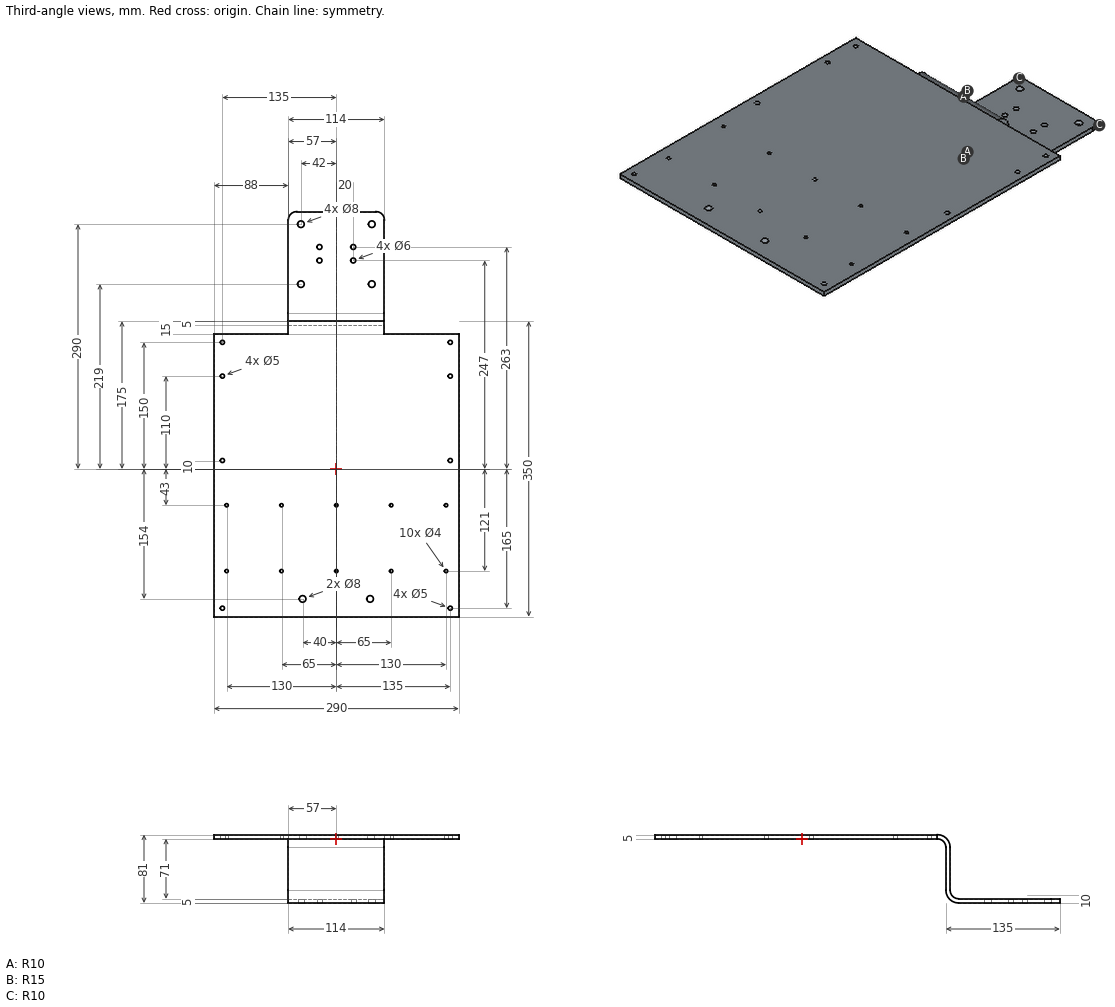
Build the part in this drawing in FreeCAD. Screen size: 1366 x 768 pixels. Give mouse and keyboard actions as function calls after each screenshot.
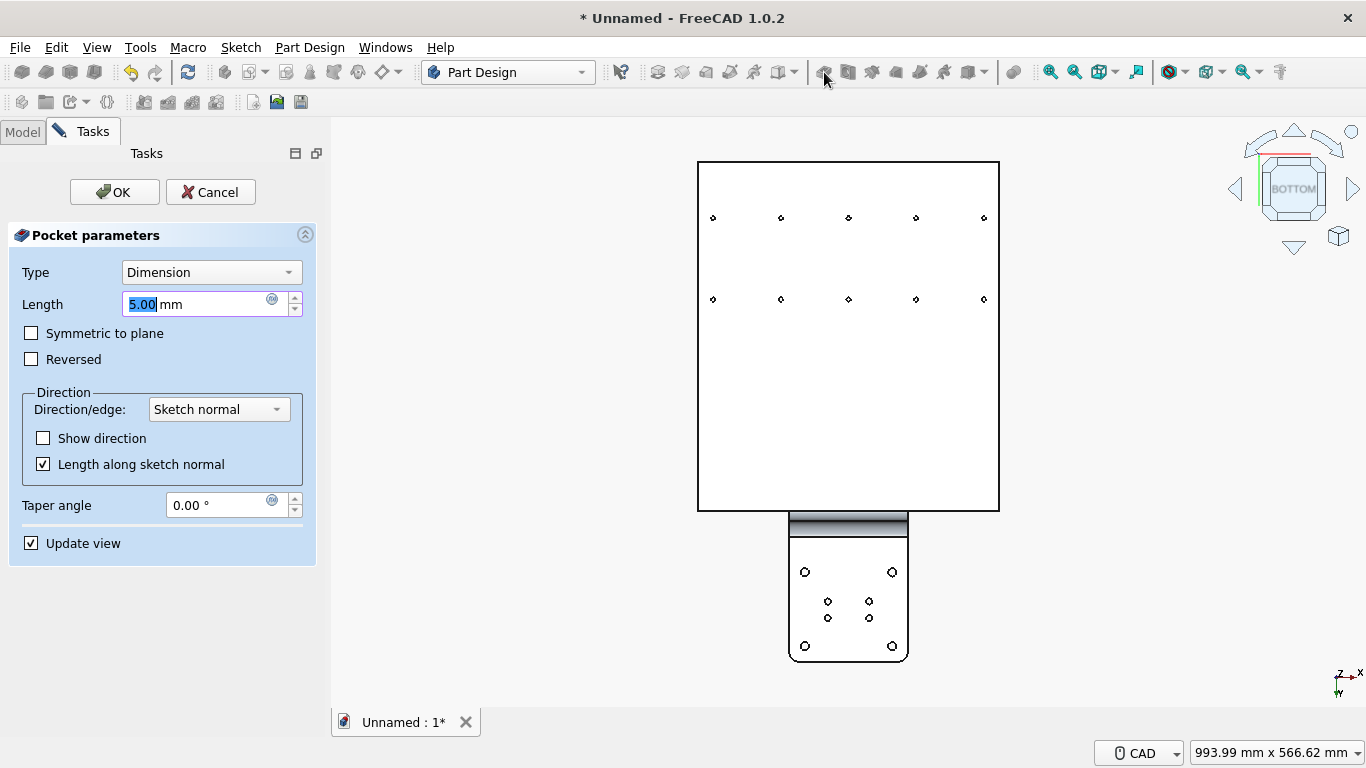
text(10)
key(Tab)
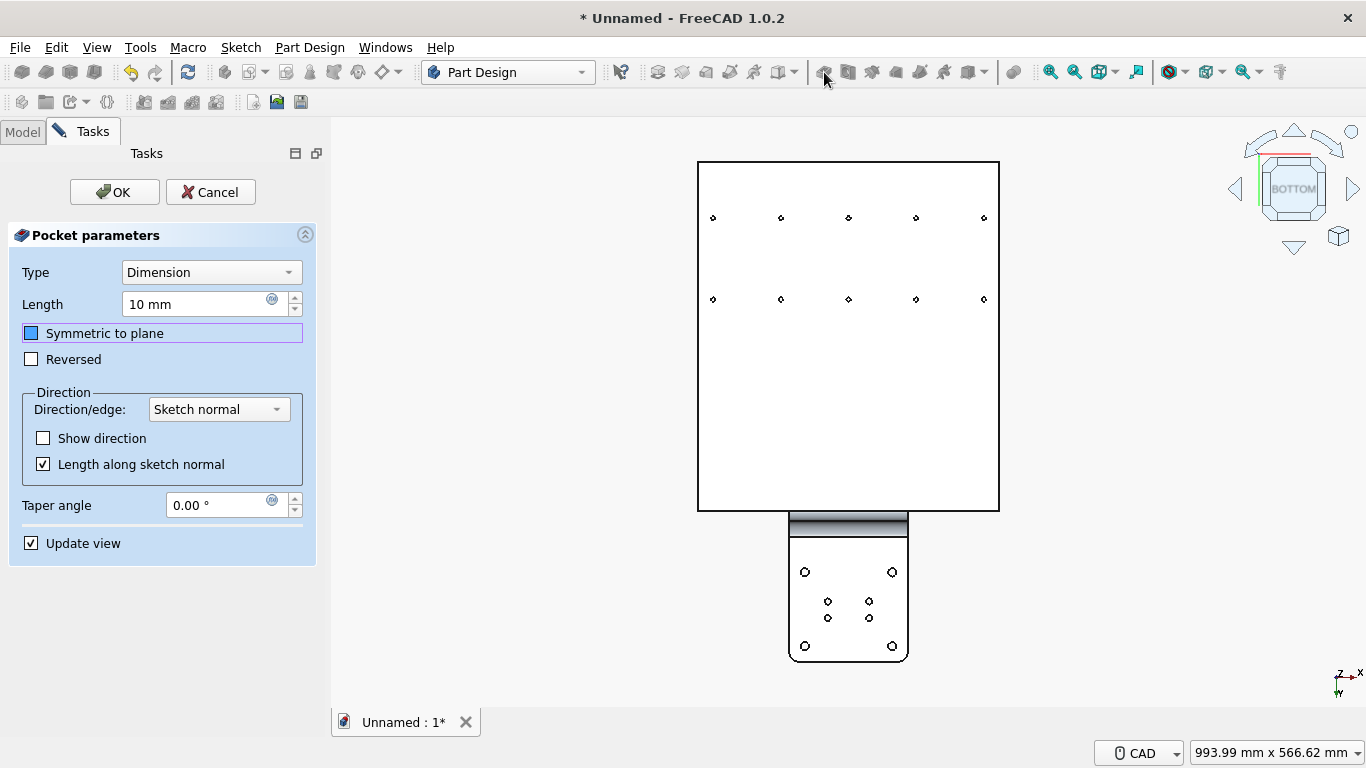
click(30, 359)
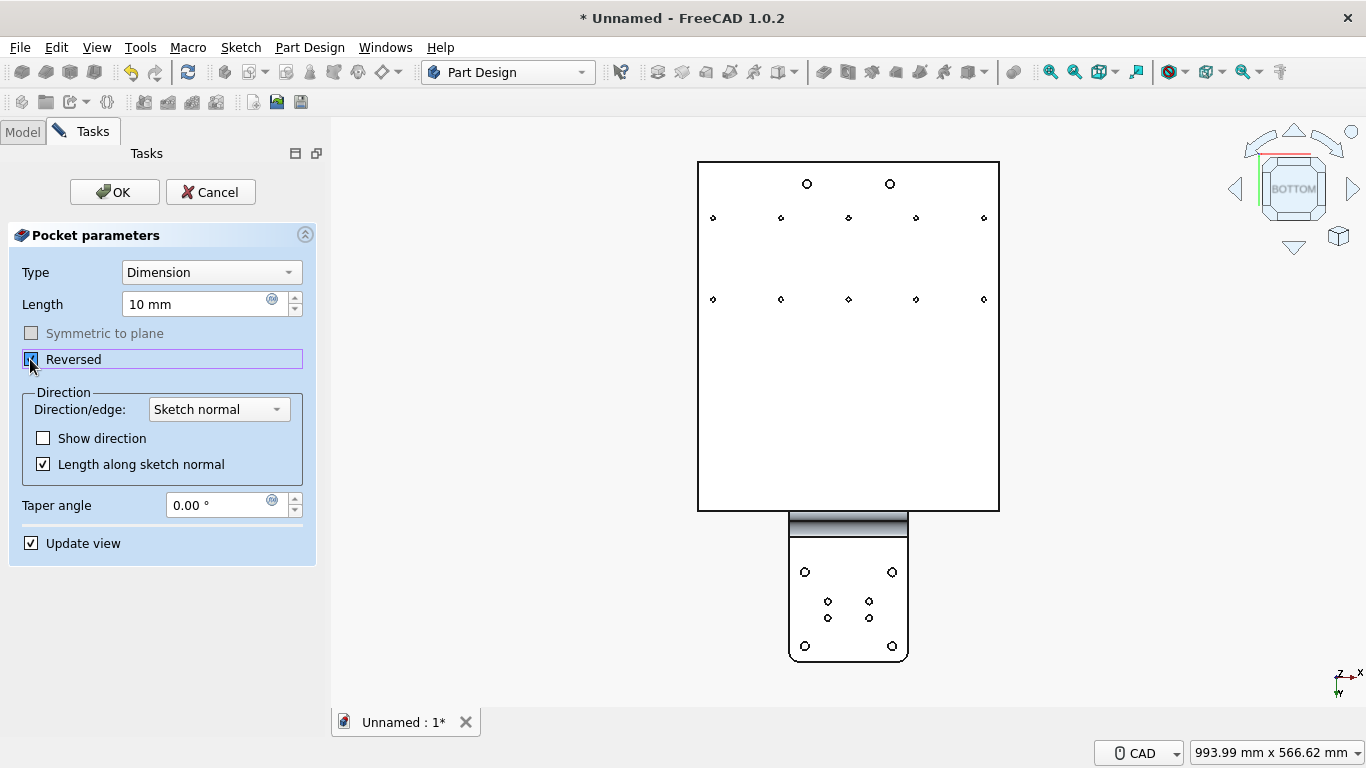
click(115, 192)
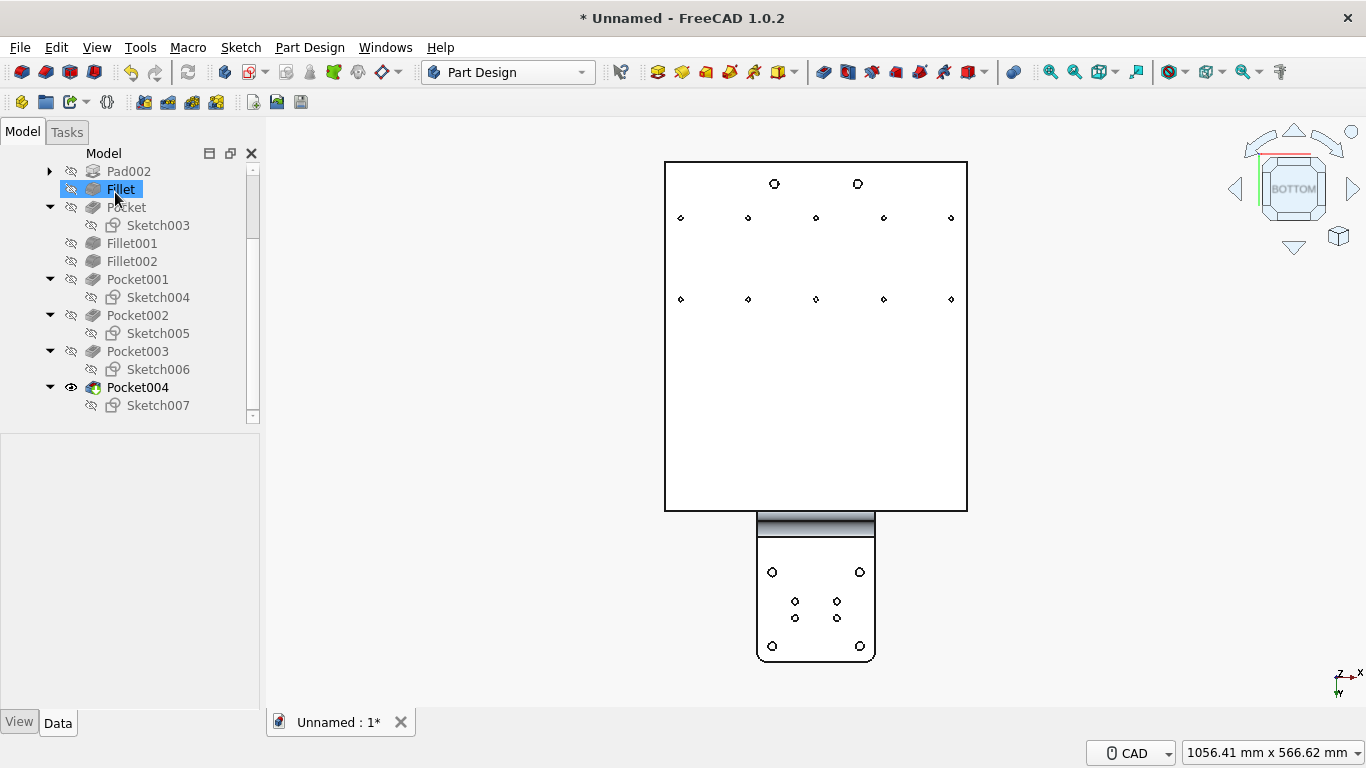
click(859, 385)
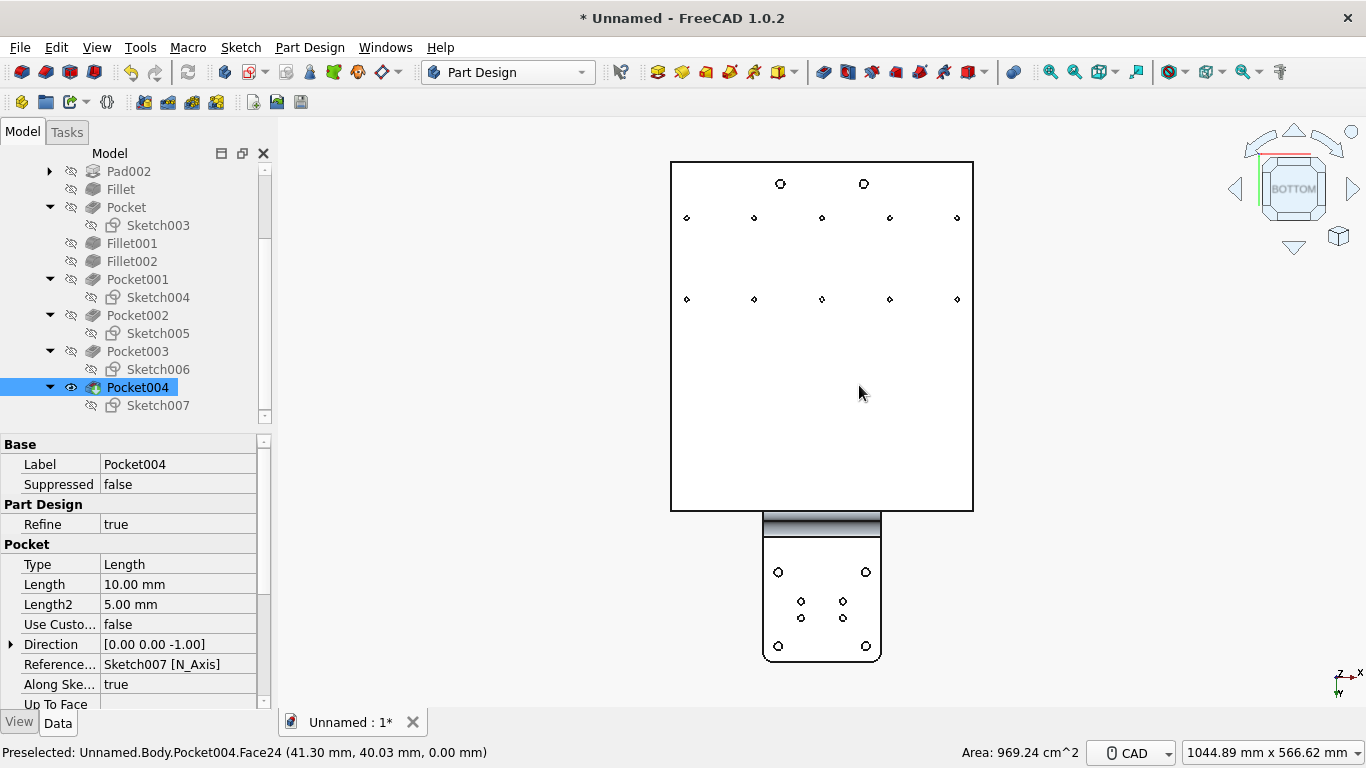
click(250, 72)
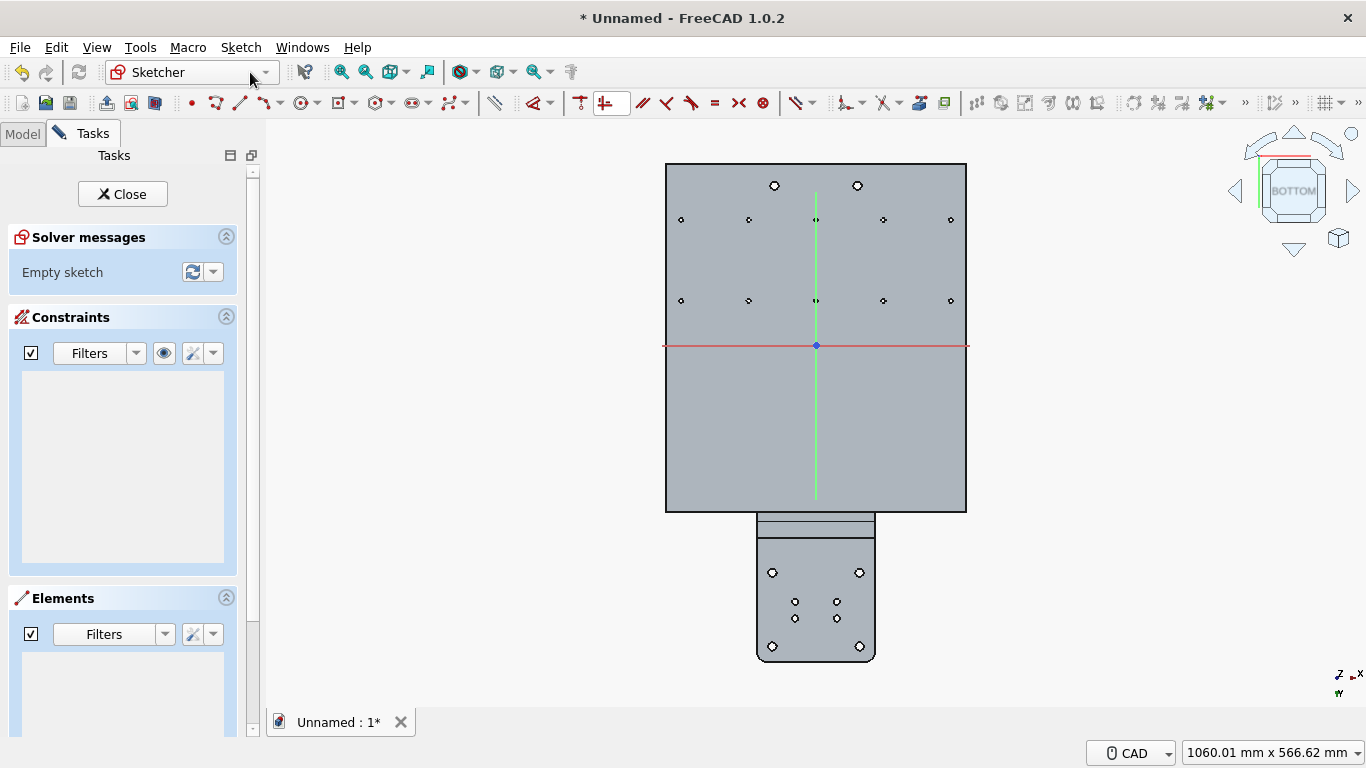
scroll(1125, 147, up, 1)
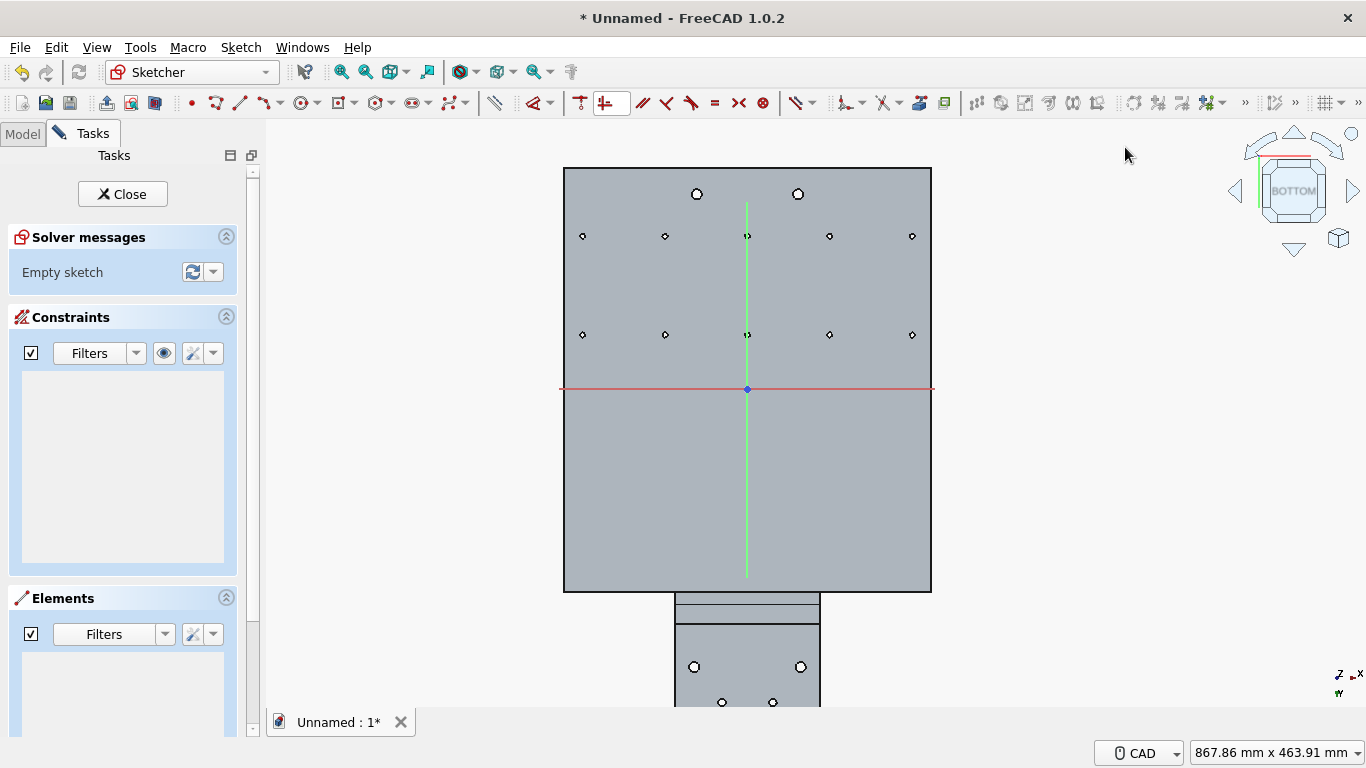
click(302, 104)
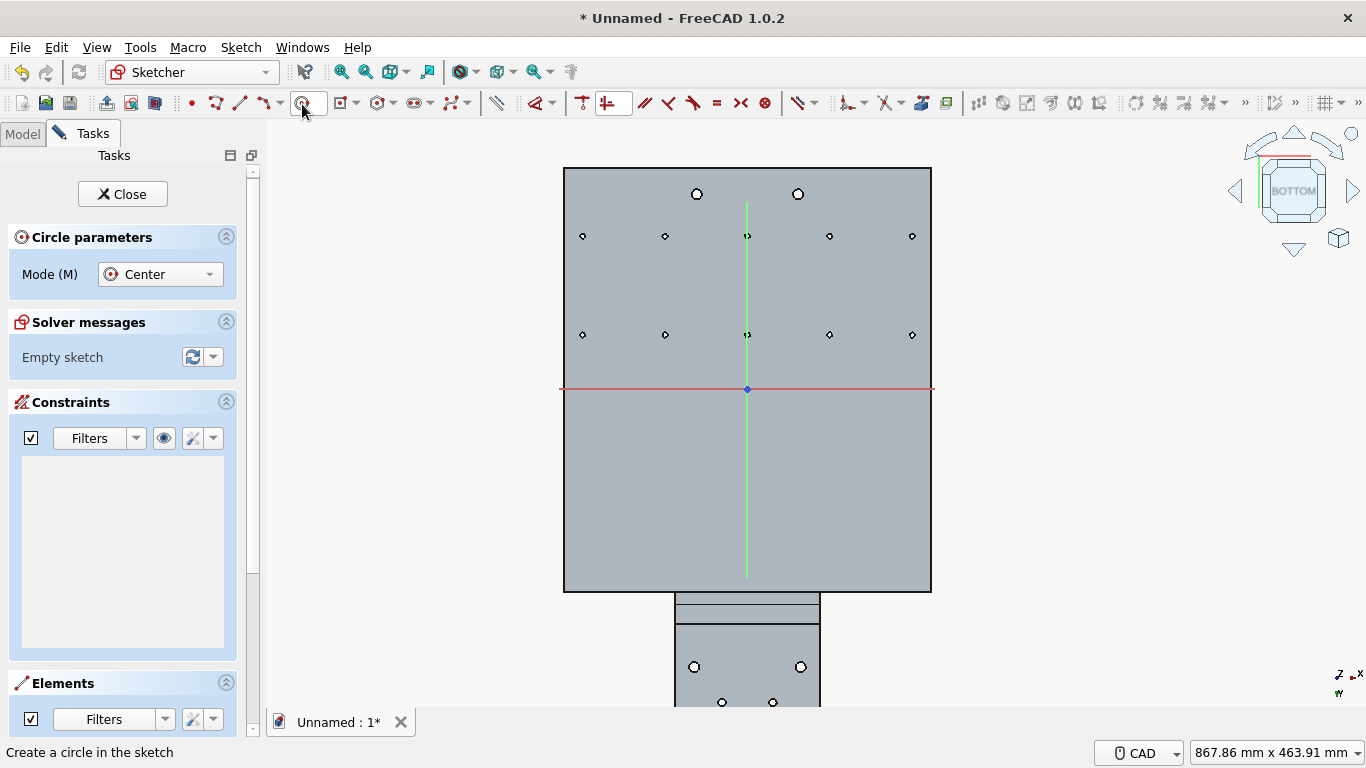
scroll(919, 180, up, 10)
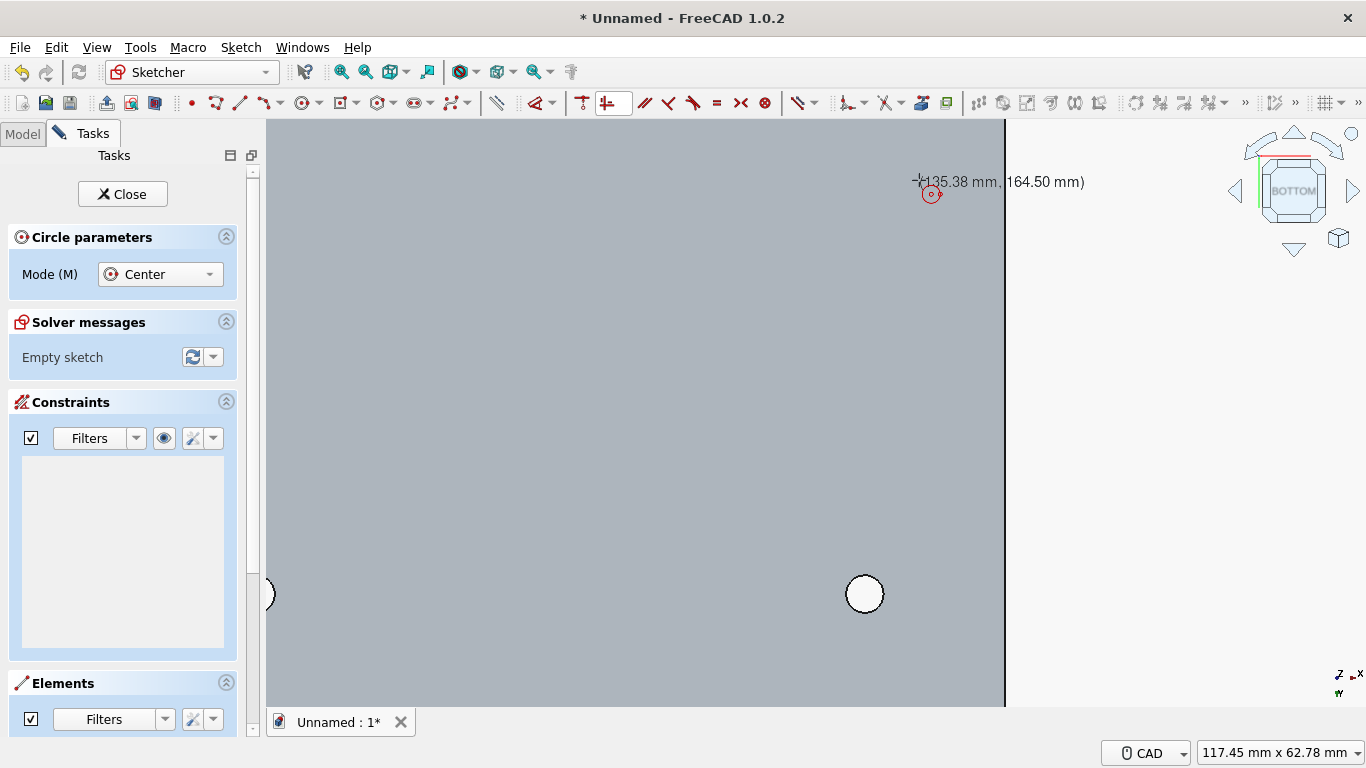
scroll(920, 218, down, 10)